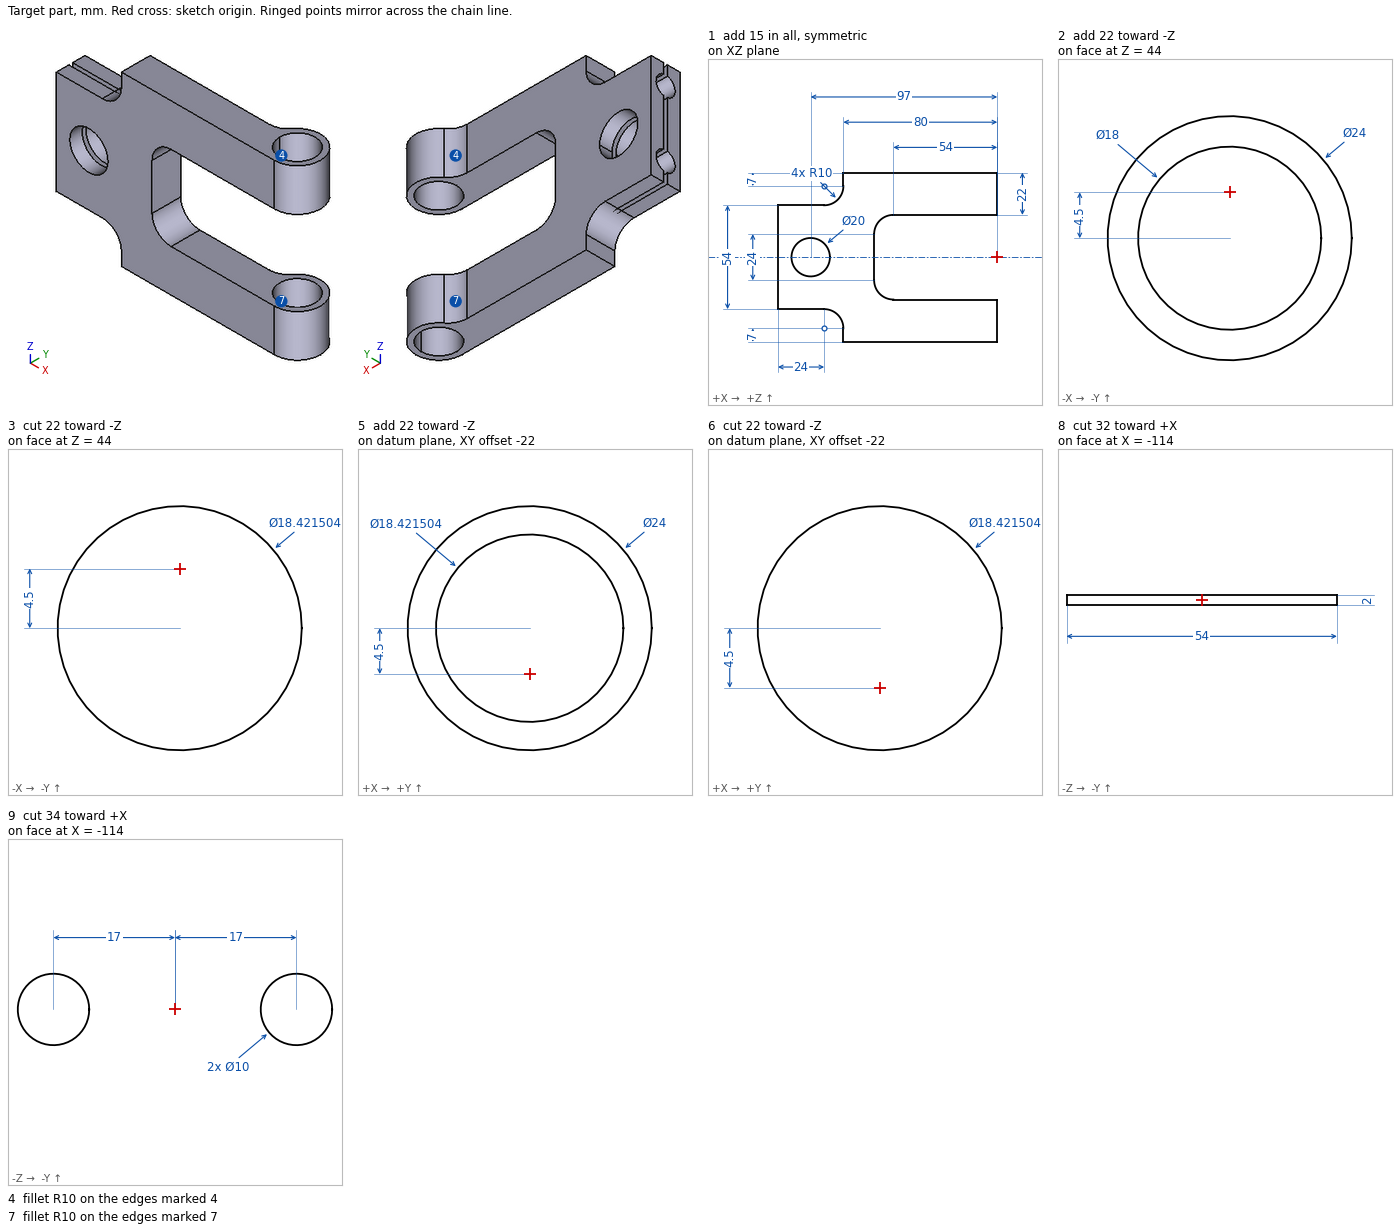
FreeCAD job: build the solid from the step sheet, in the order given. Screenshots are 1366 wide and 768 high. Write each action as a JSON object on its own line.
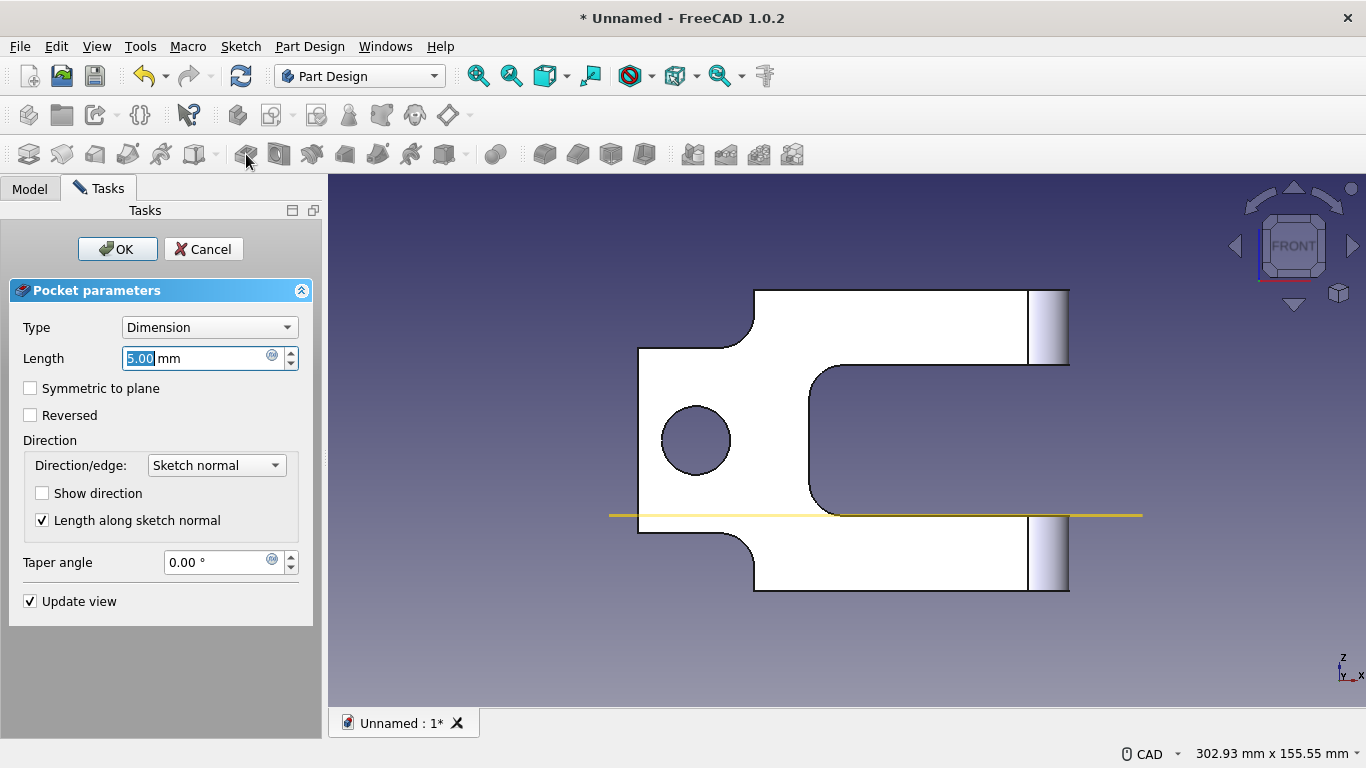
{"action": "type", "text": "22"}
{"action": "key", "text": "Tab"}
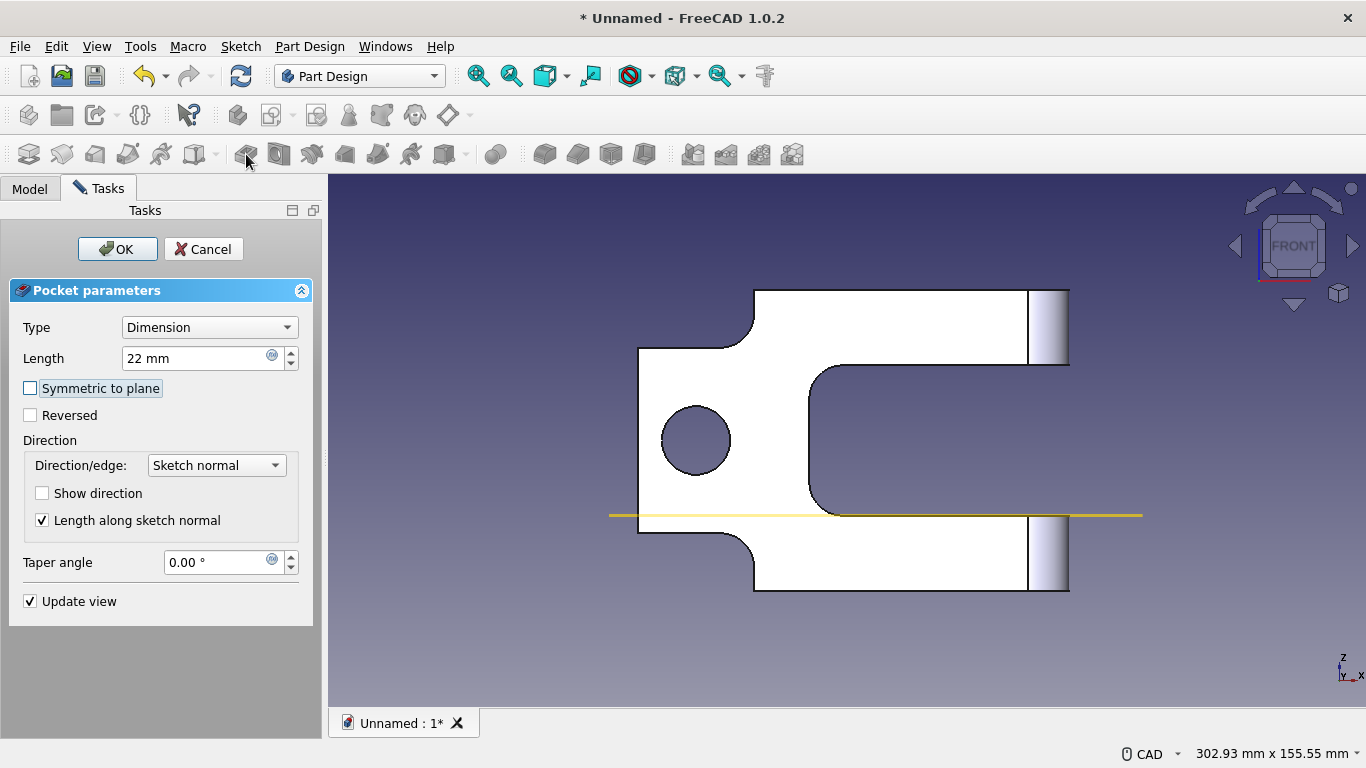
{"action": "left_click", "coordinate": [118, 249]}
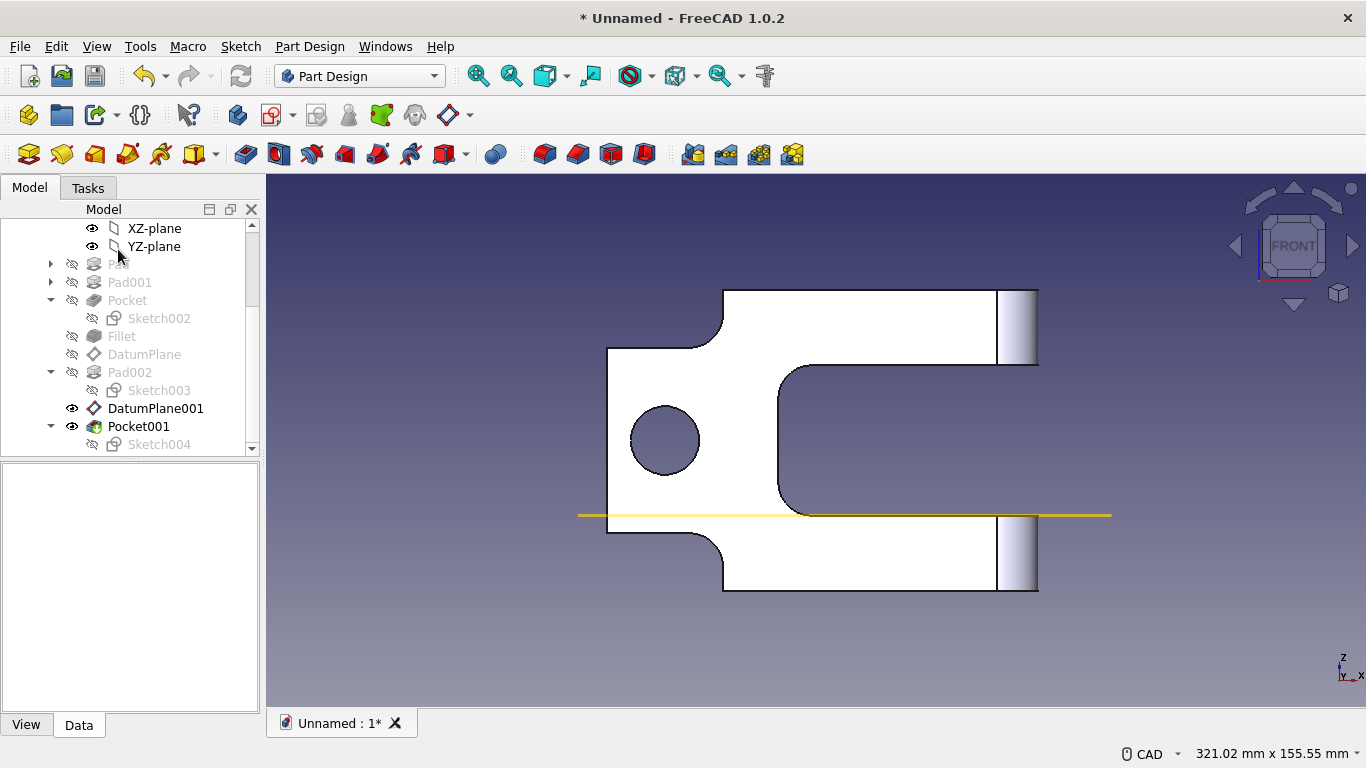
{"action": "left_click", "coordinate": [117, 408]}
{"action": "key", "text": "space"}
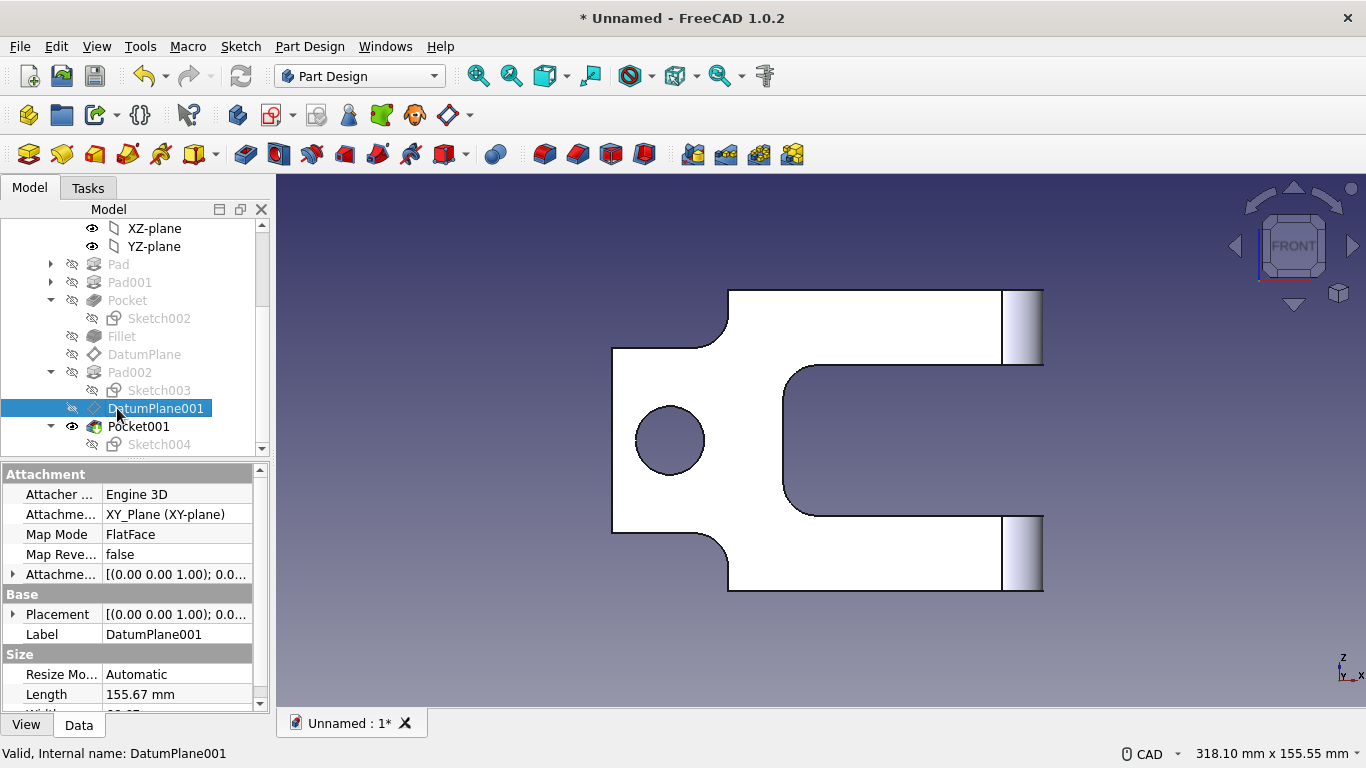
{"action": "key", "text": "0"}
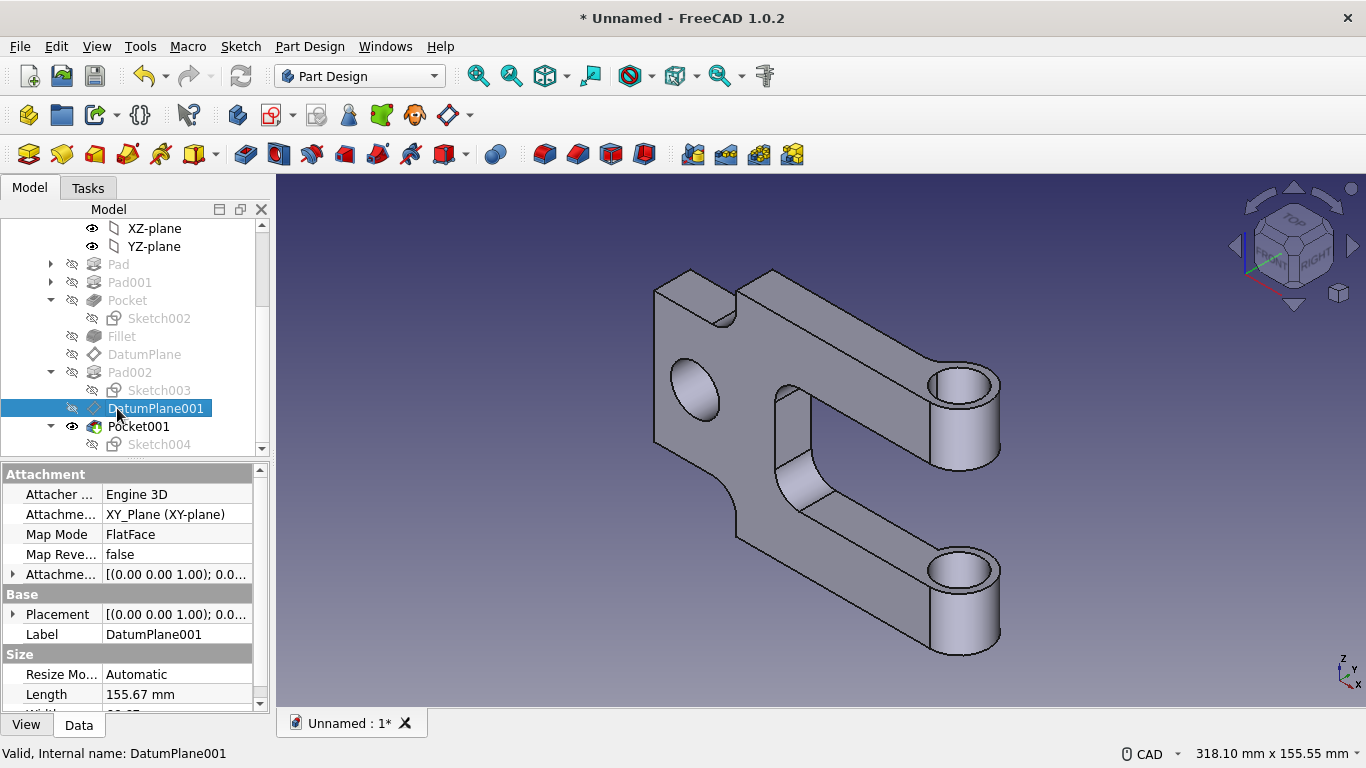
{"action": "key", "text": "2"}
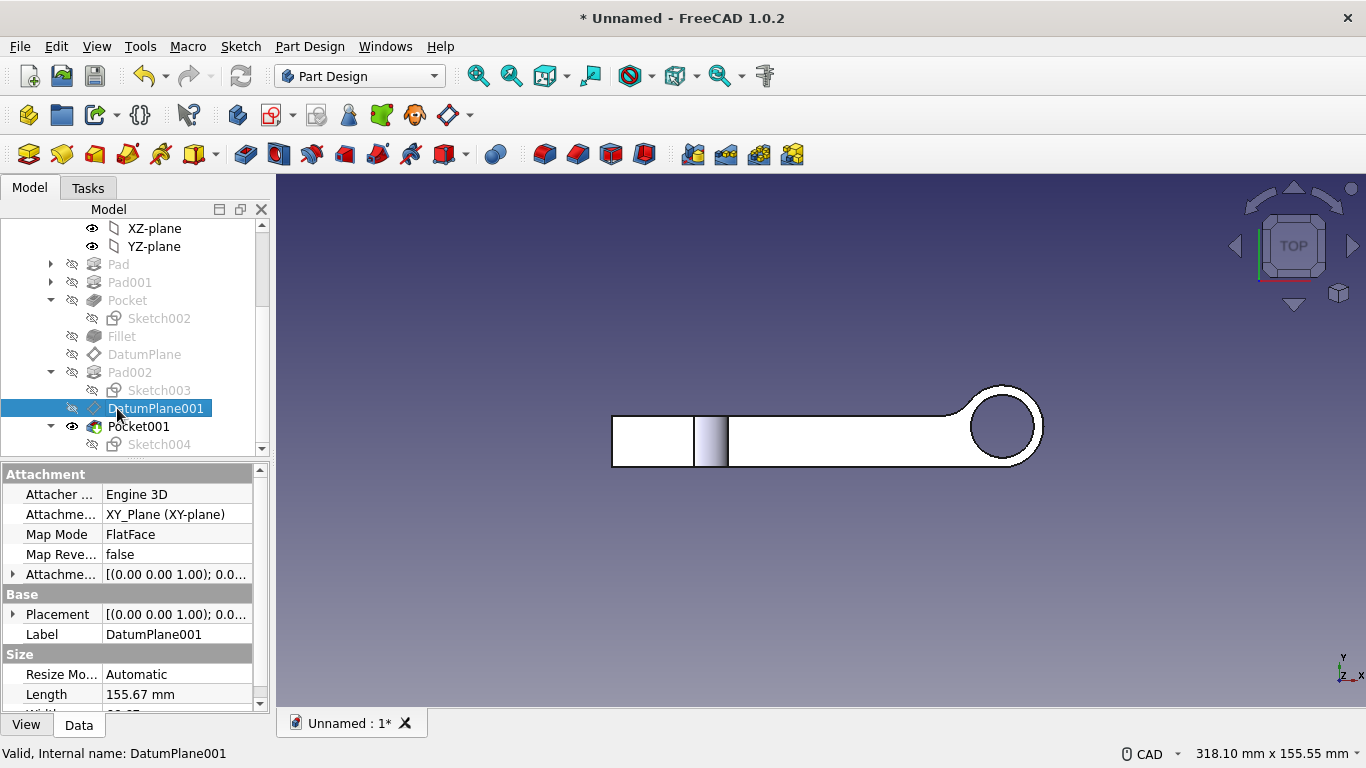
{"action": "left_click", "coordinate": [479, 76]}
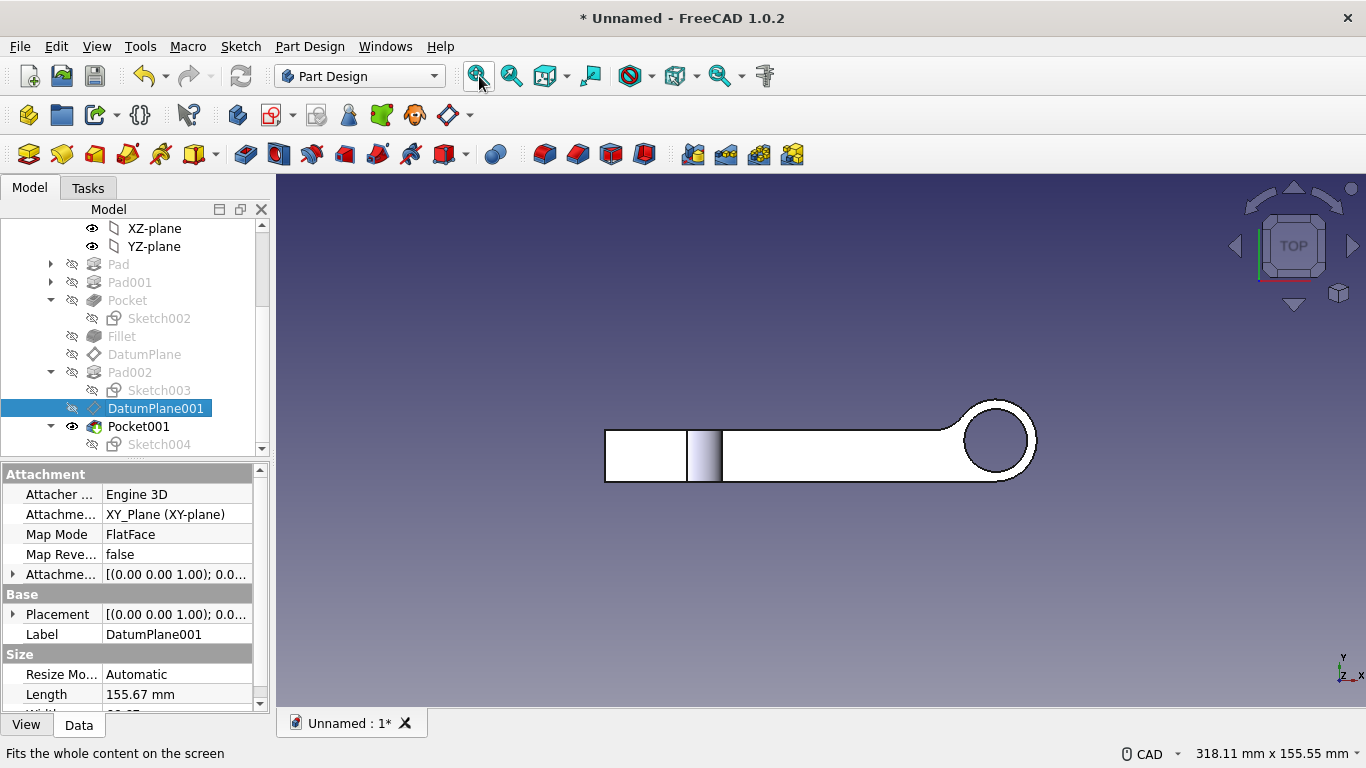
{"action": "key", "text": "1"}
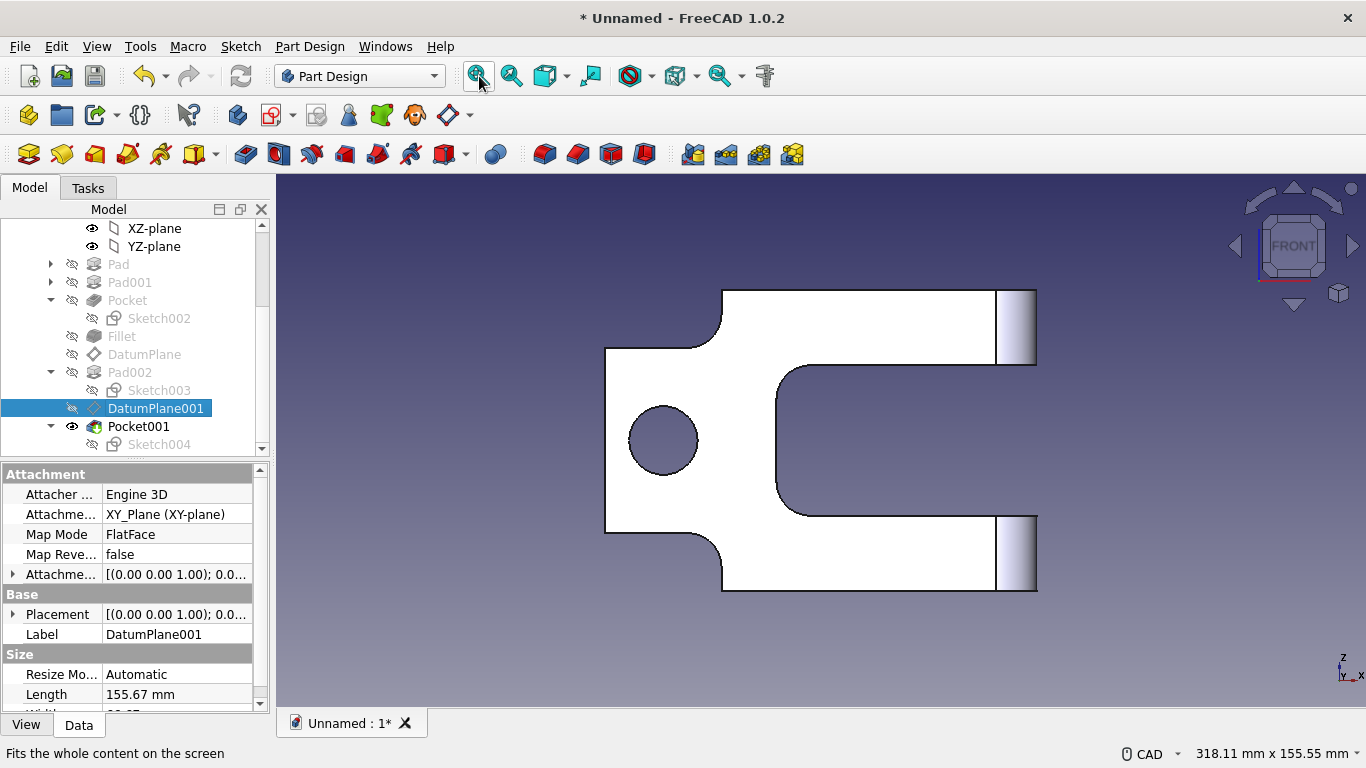
{"action": "key", "text": "3"}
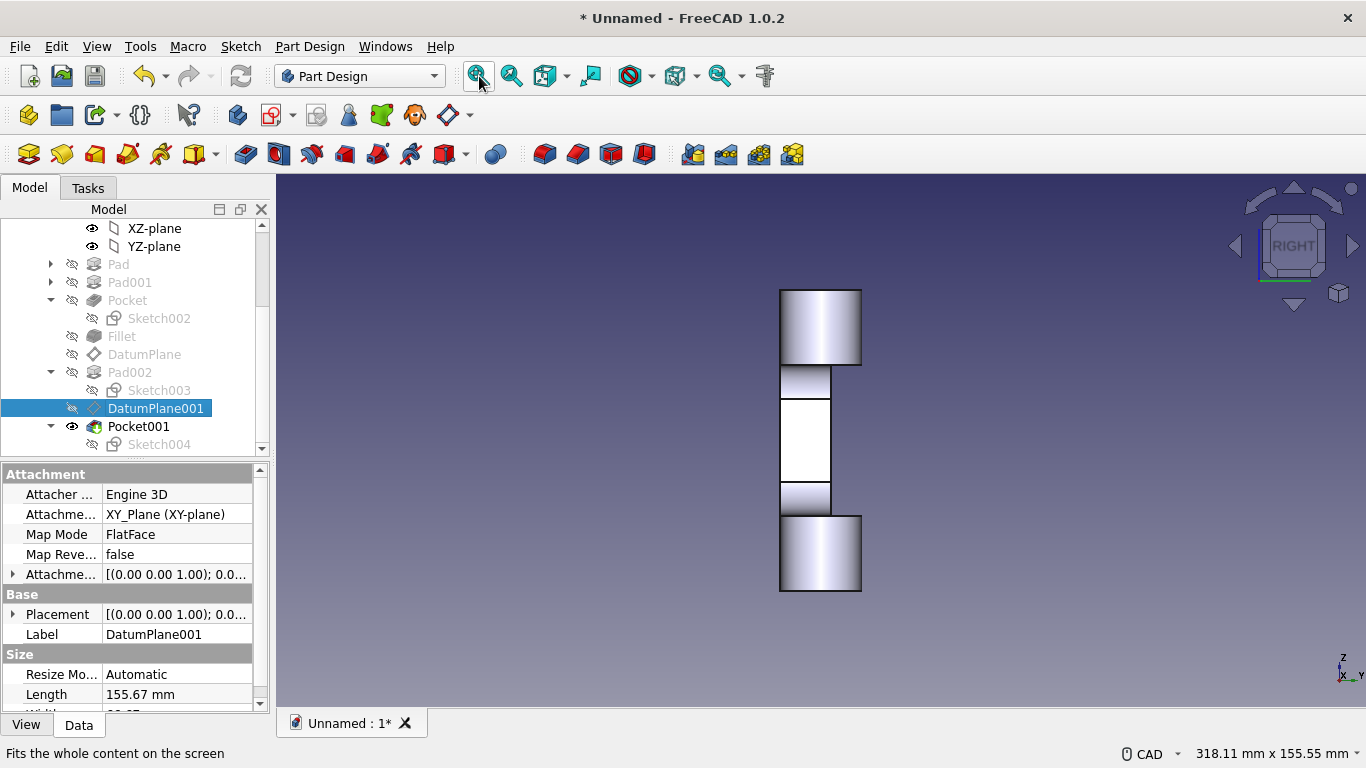
{"action": "key", "text": "5"}